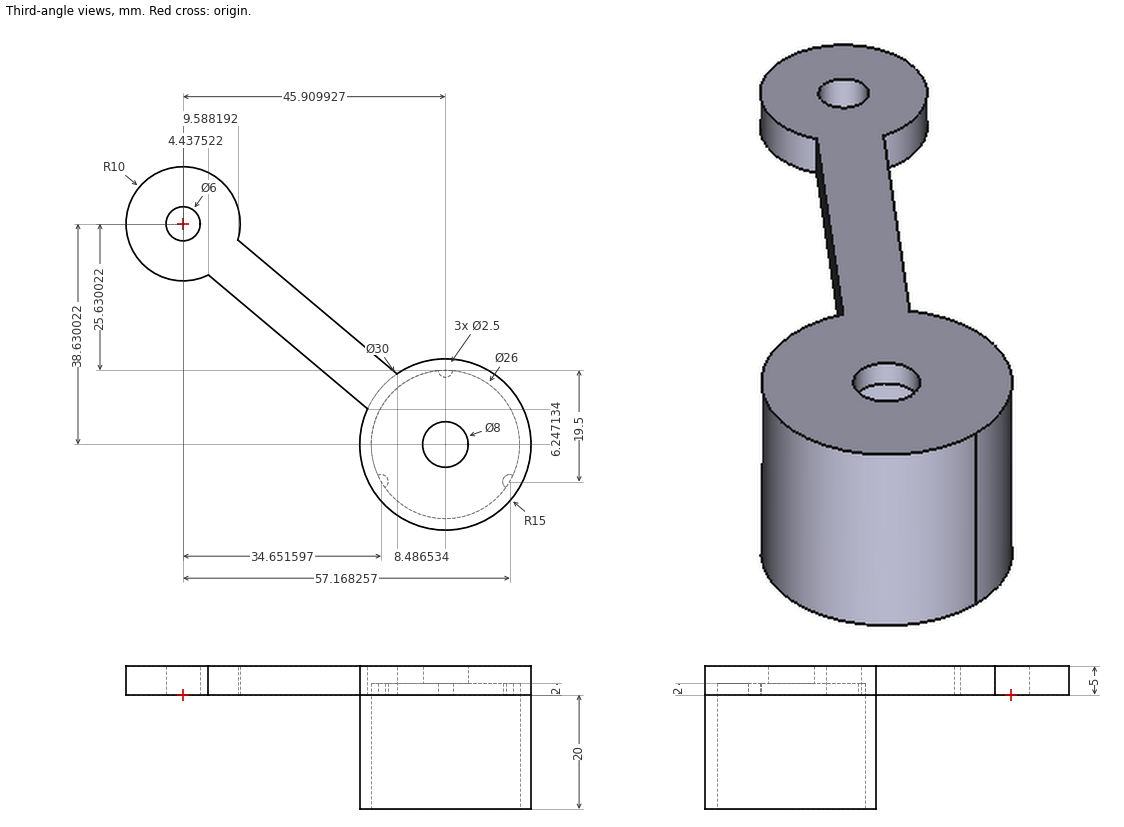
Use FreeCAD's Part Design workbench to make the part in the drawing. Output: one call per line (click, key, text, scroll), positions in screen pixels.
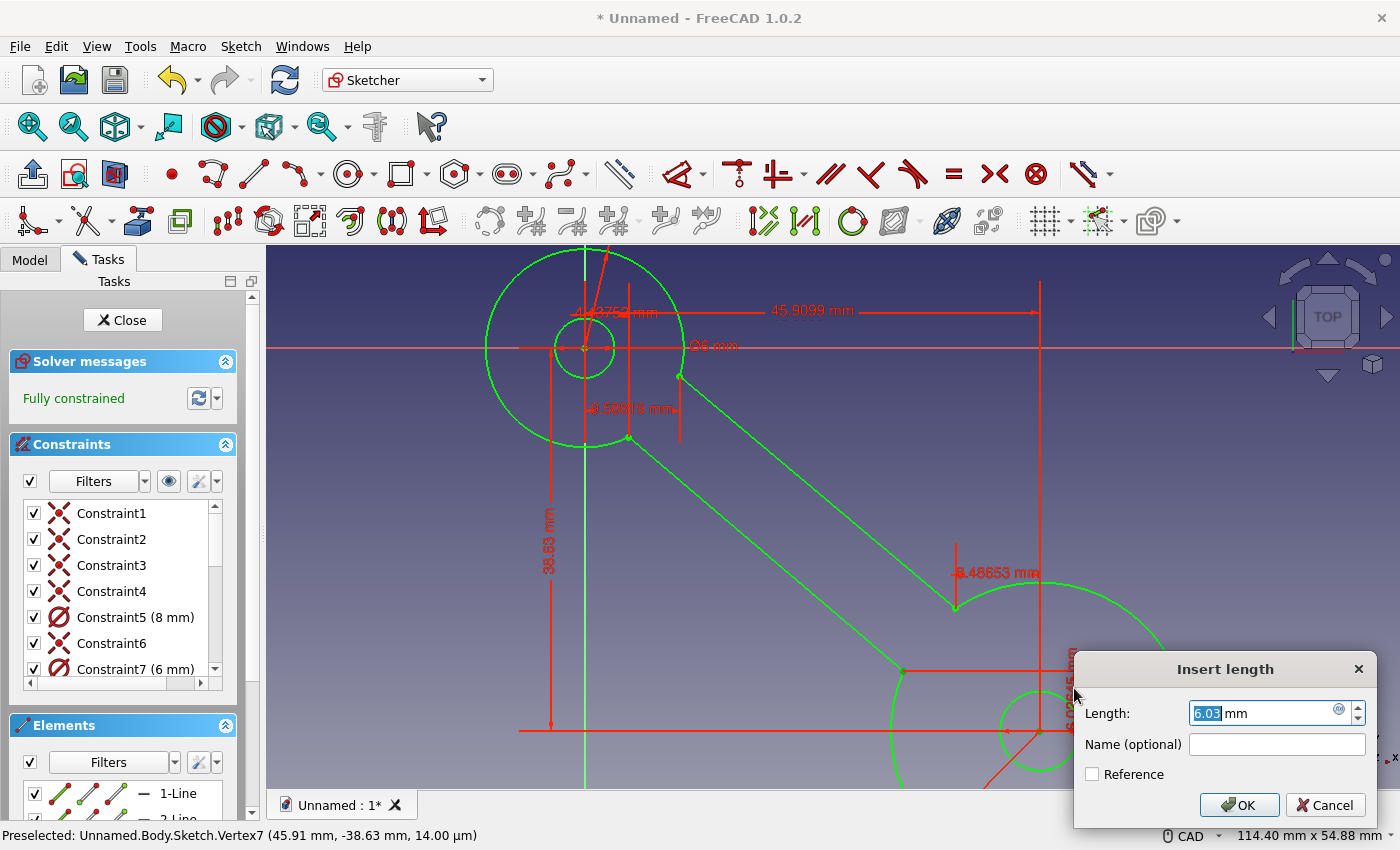
text(6.247134)
key(Return)
key(Escape)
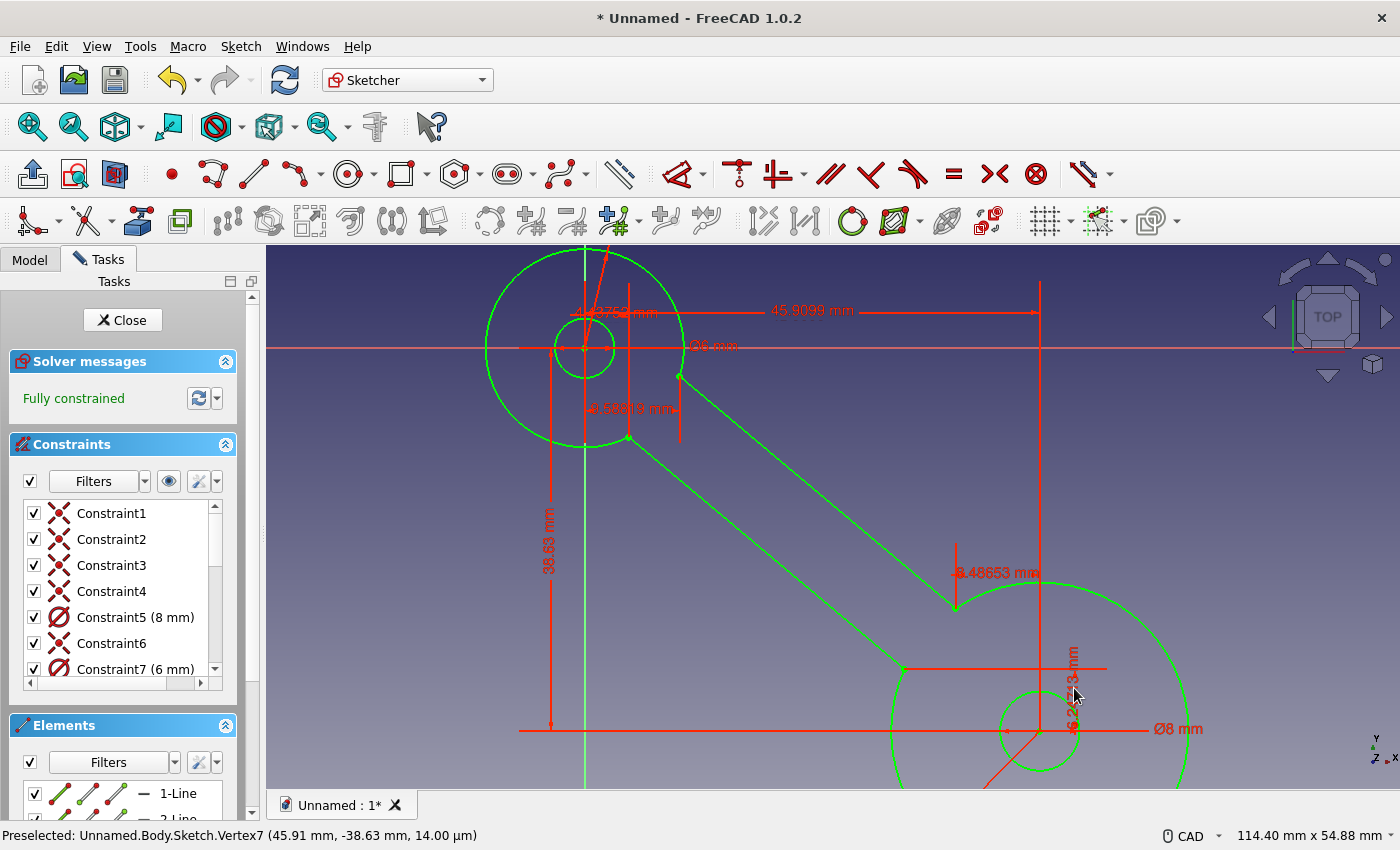
click(123, 320)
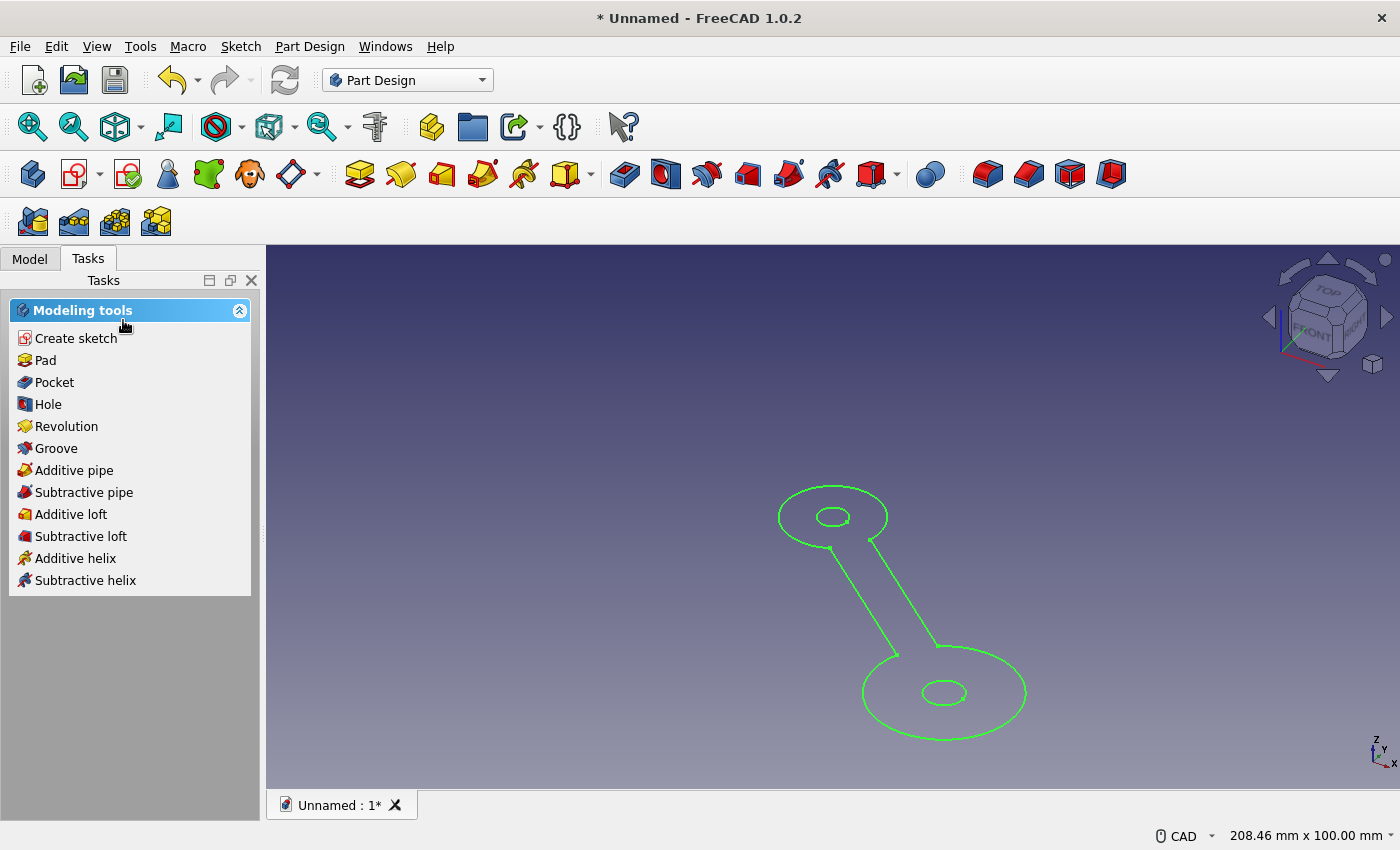
click(360, 174)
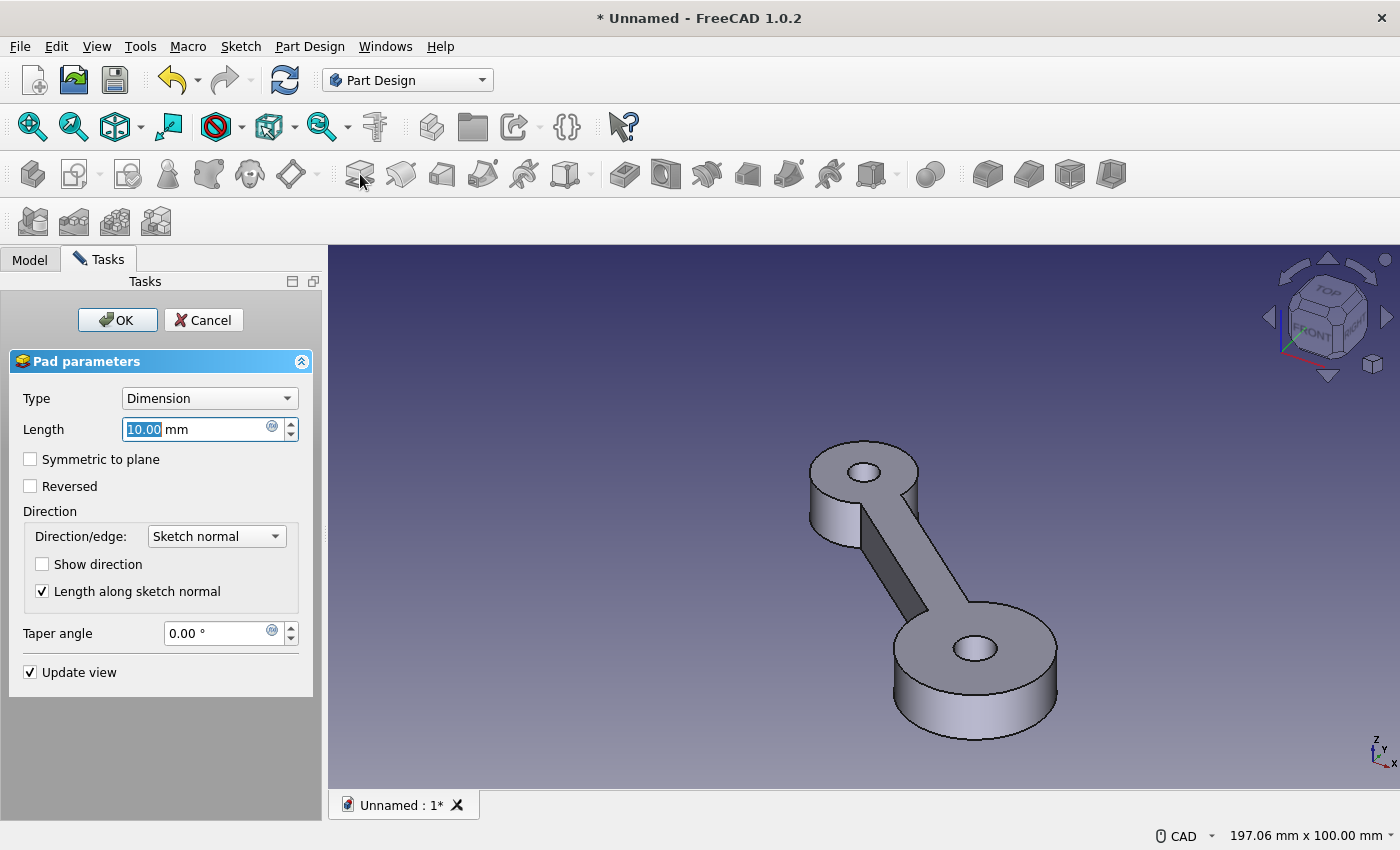
text(5)
key(Tab)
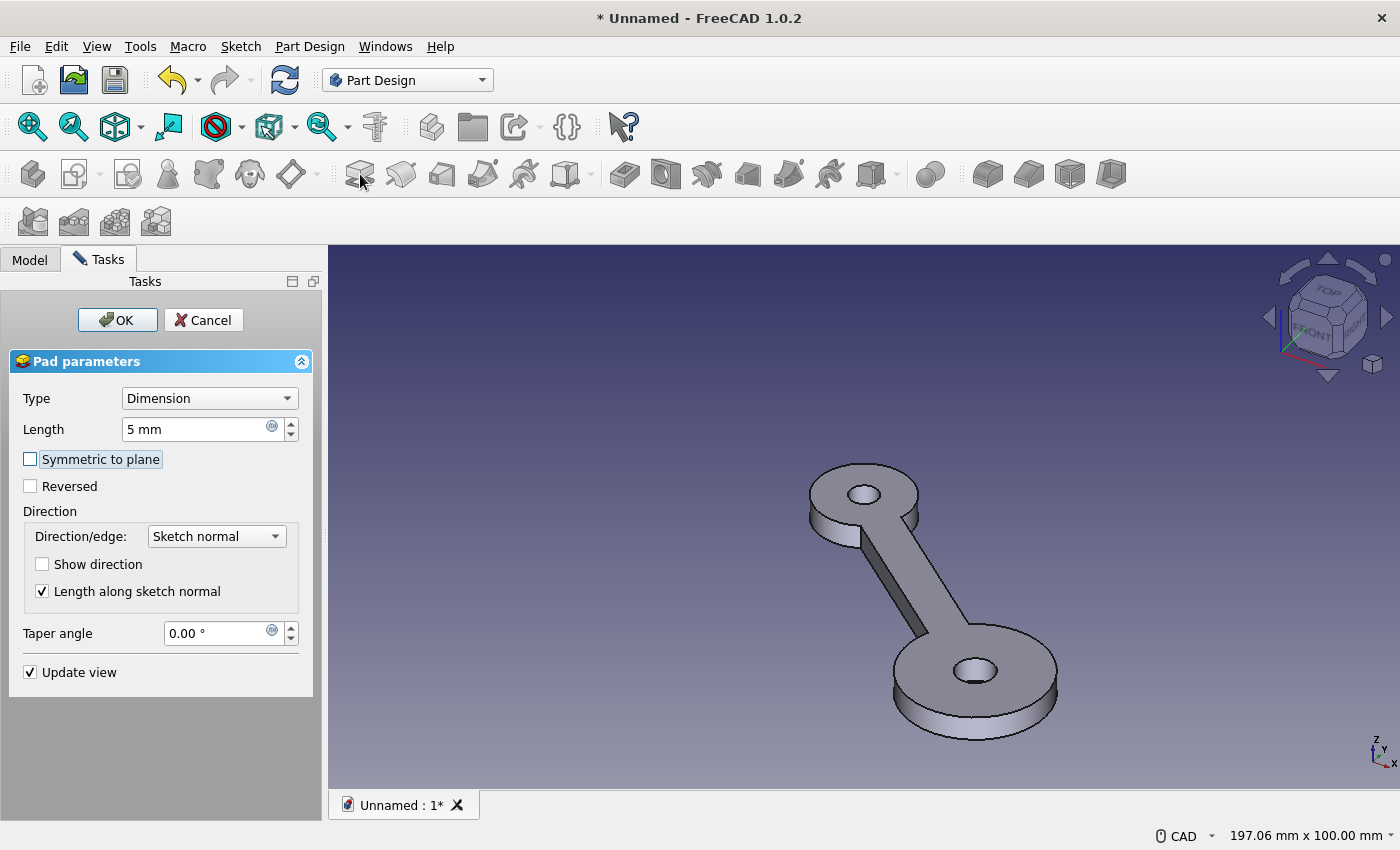
click(118, 320)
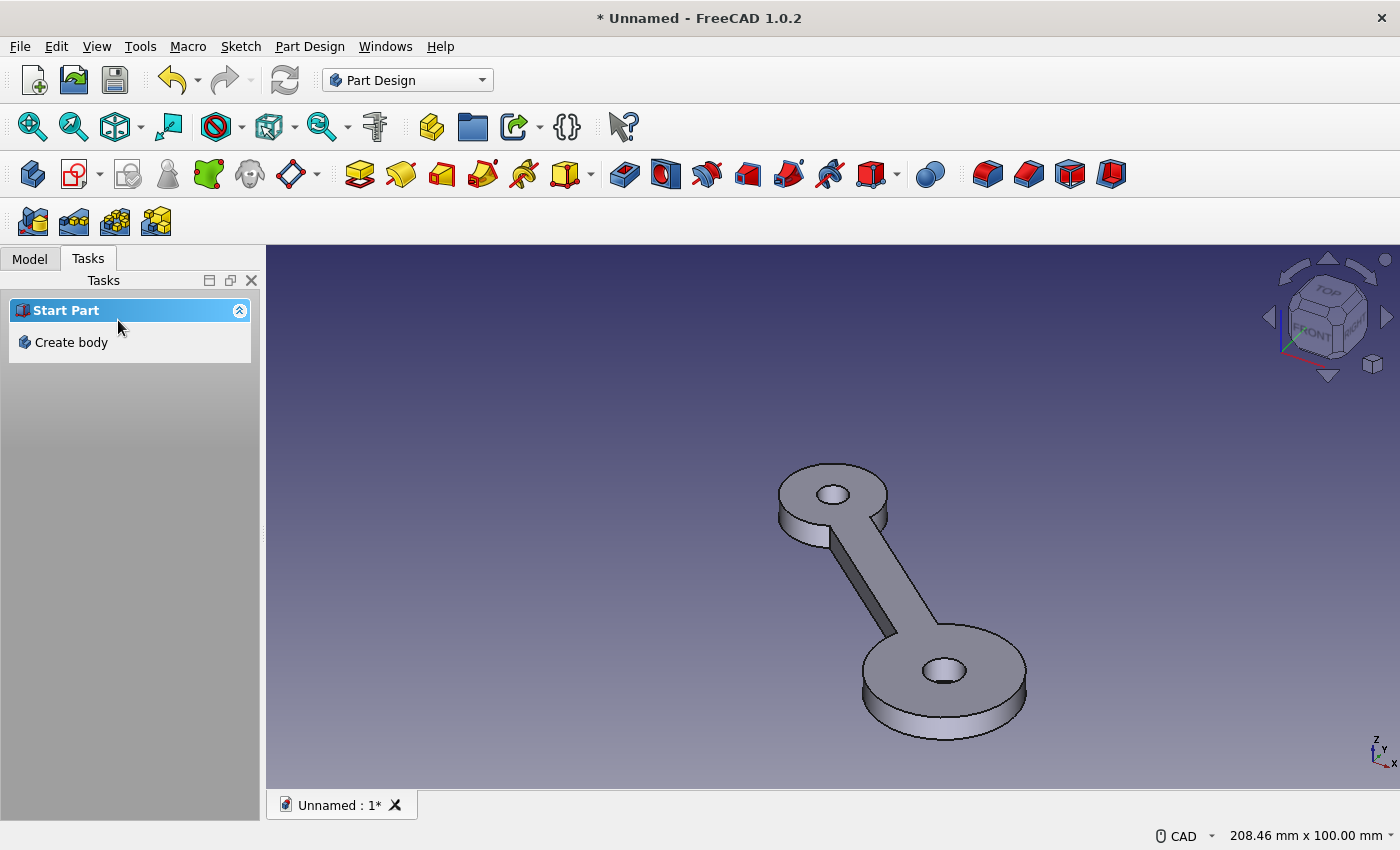
key(5)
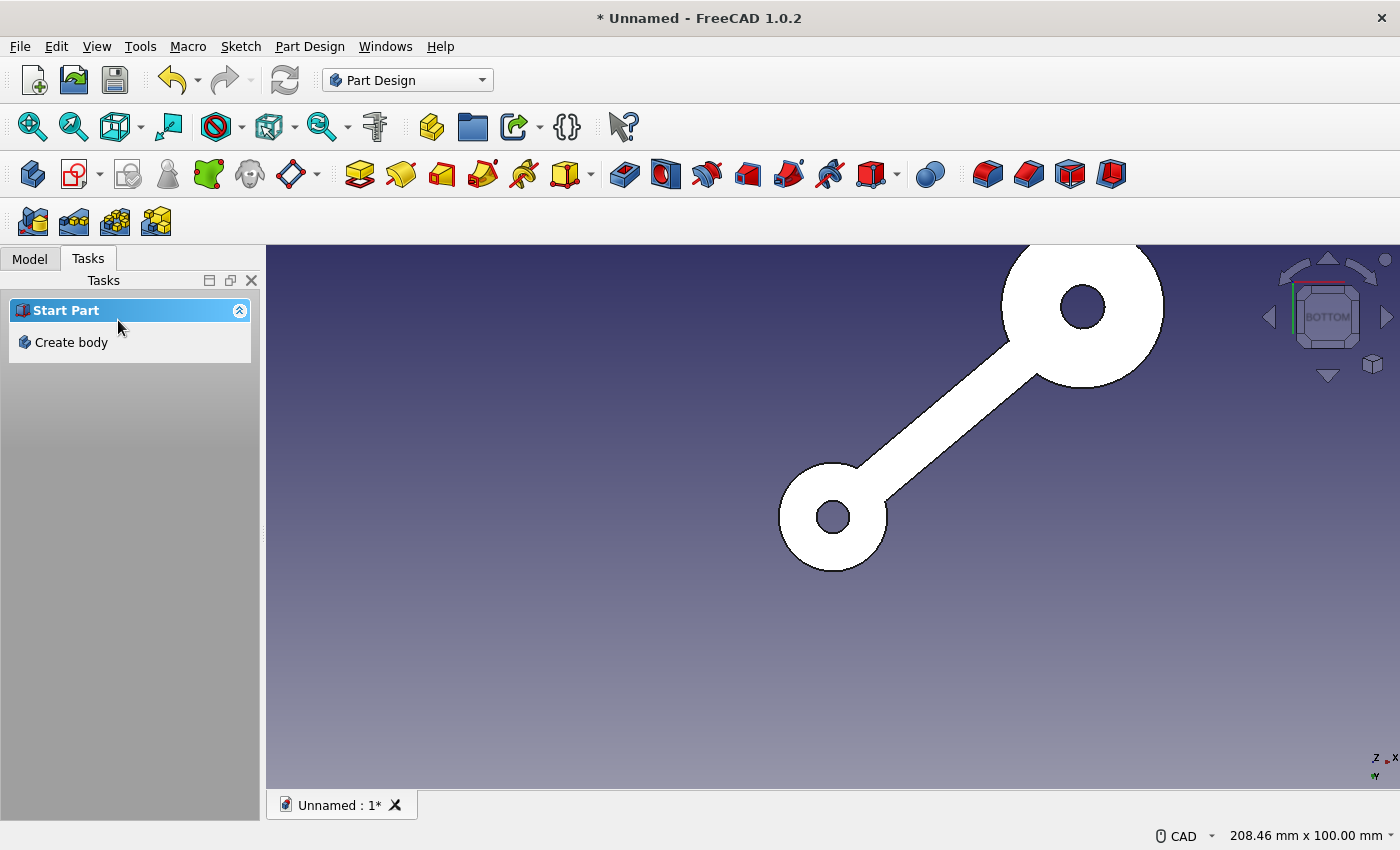
click(33, 128)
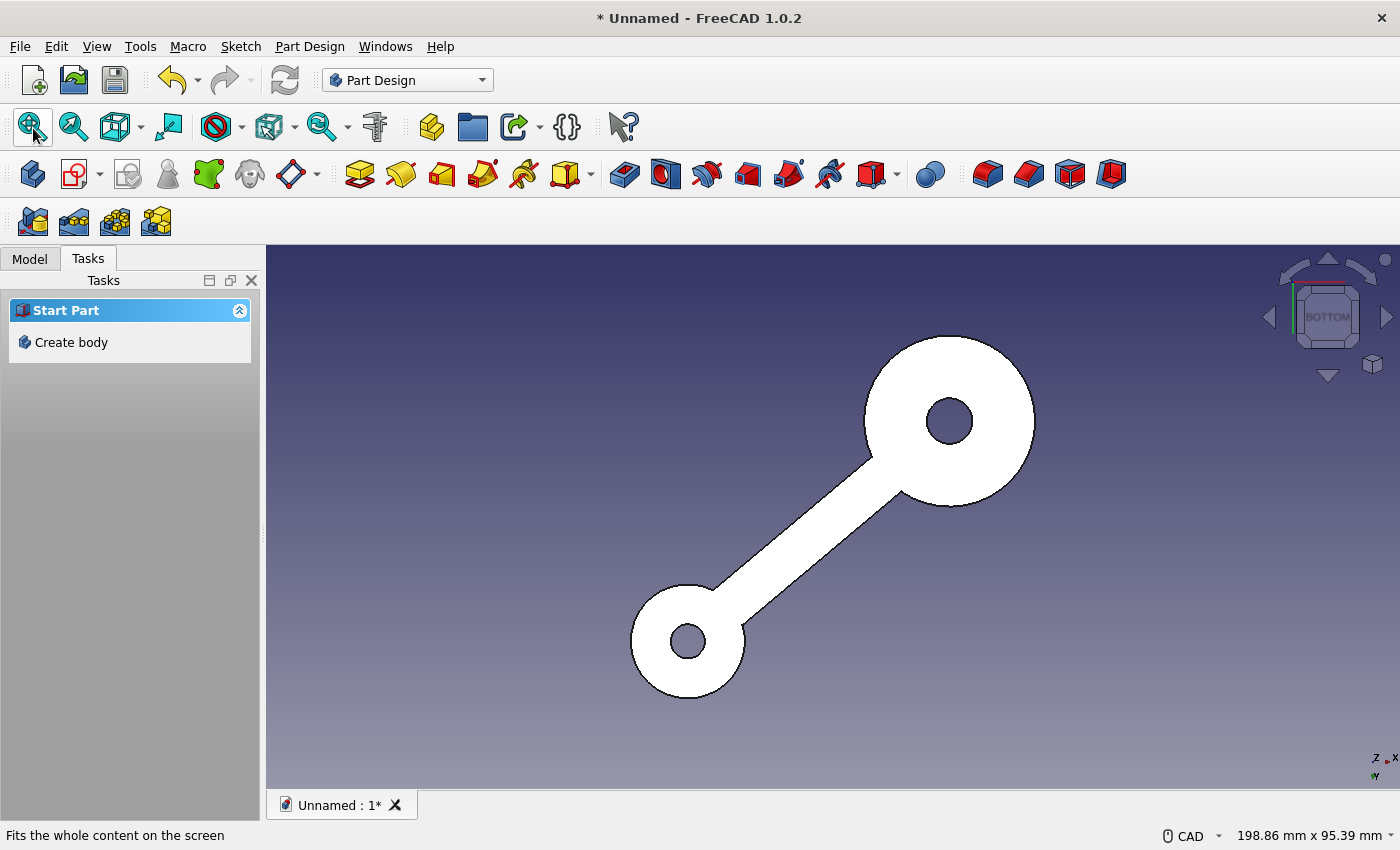
click(1006, 412)